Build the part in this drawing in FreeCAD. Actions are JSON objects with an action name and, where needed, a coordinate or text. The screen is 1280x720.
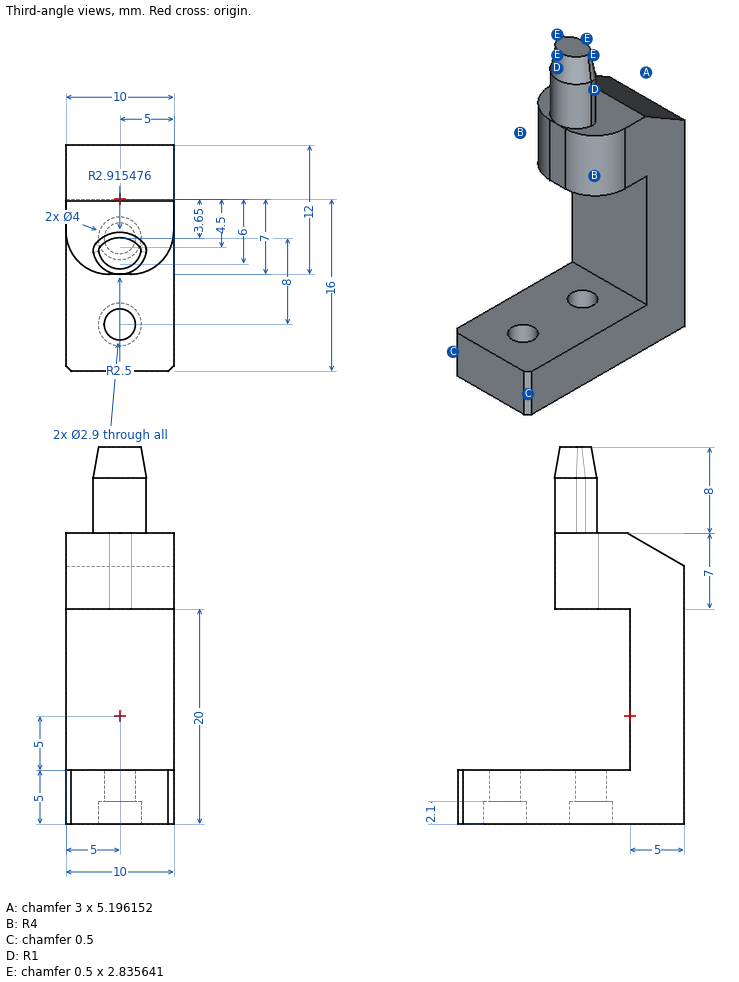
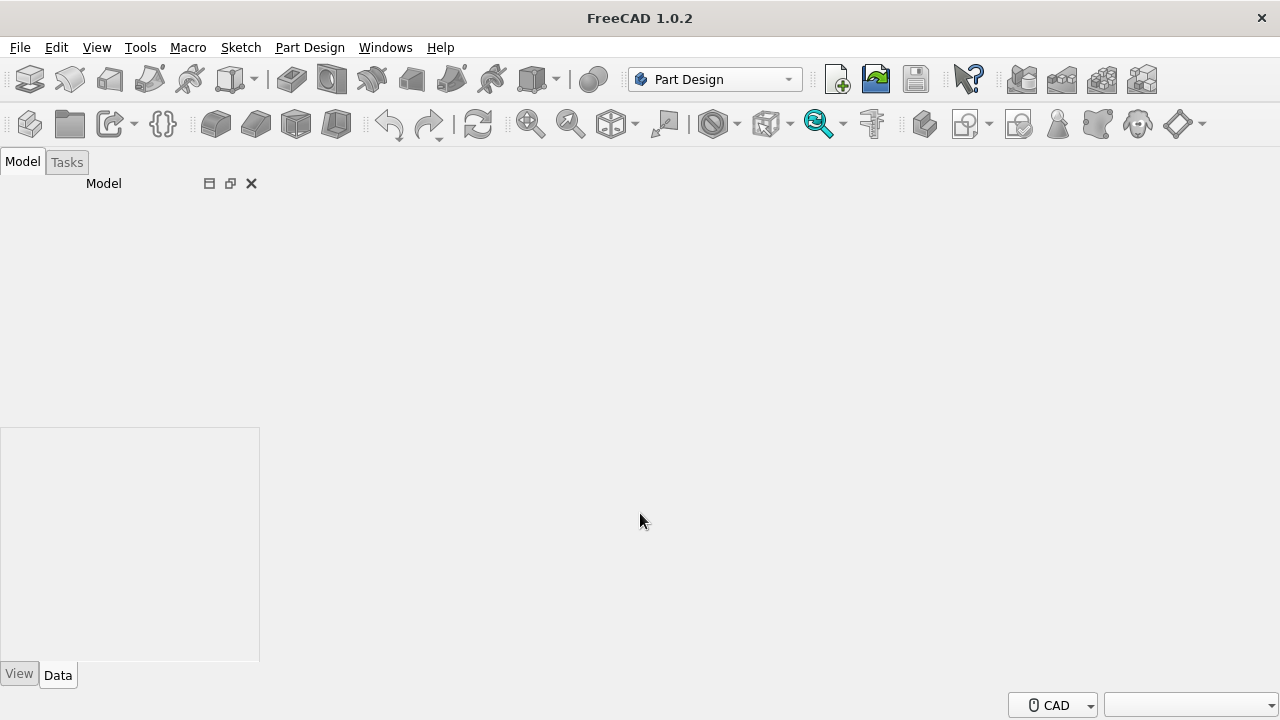
{"action": "key", "text": "ctrl+n"}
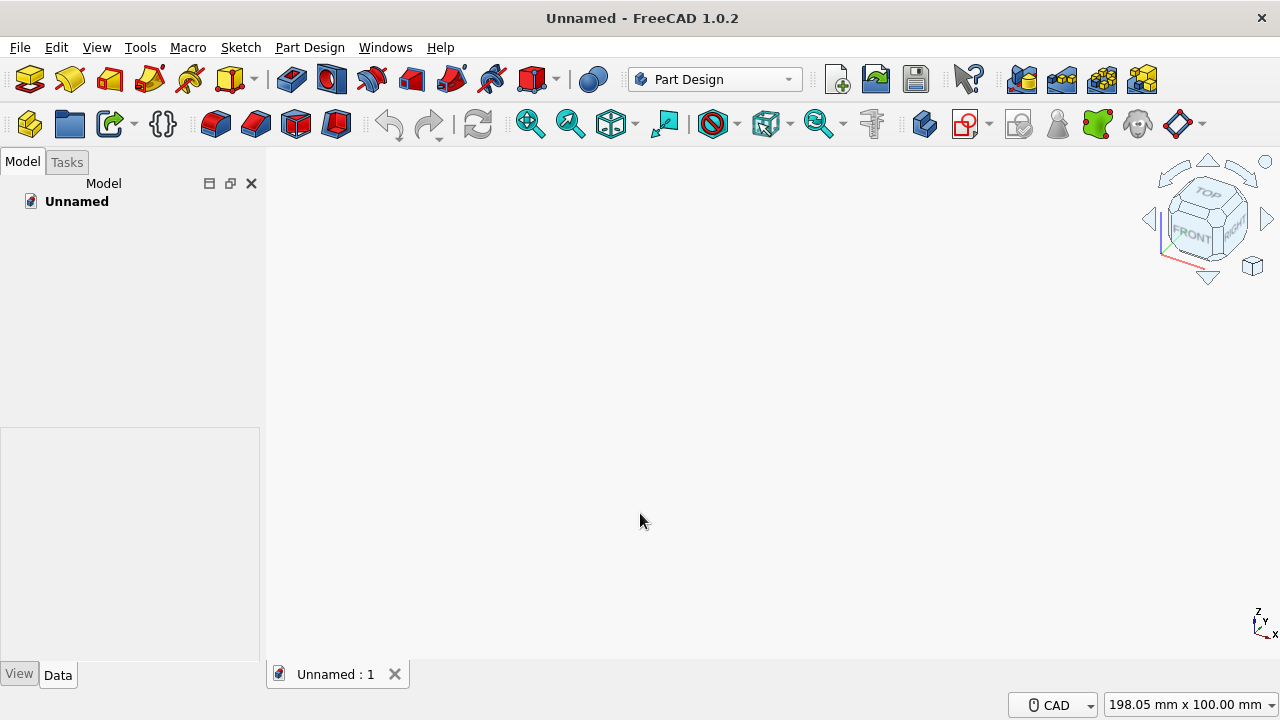
{"action": "left_click", "coordinate": [966, 124]}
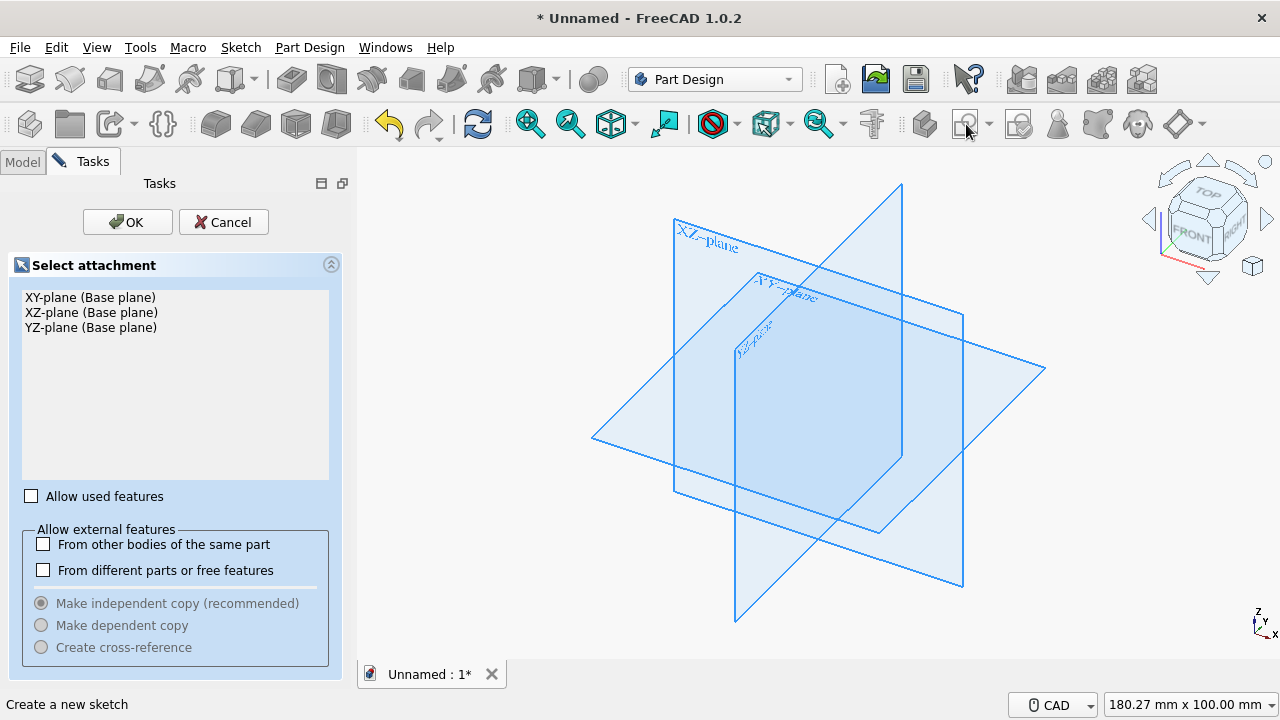
{"action": "left_click", "coordinate": [82, 312]}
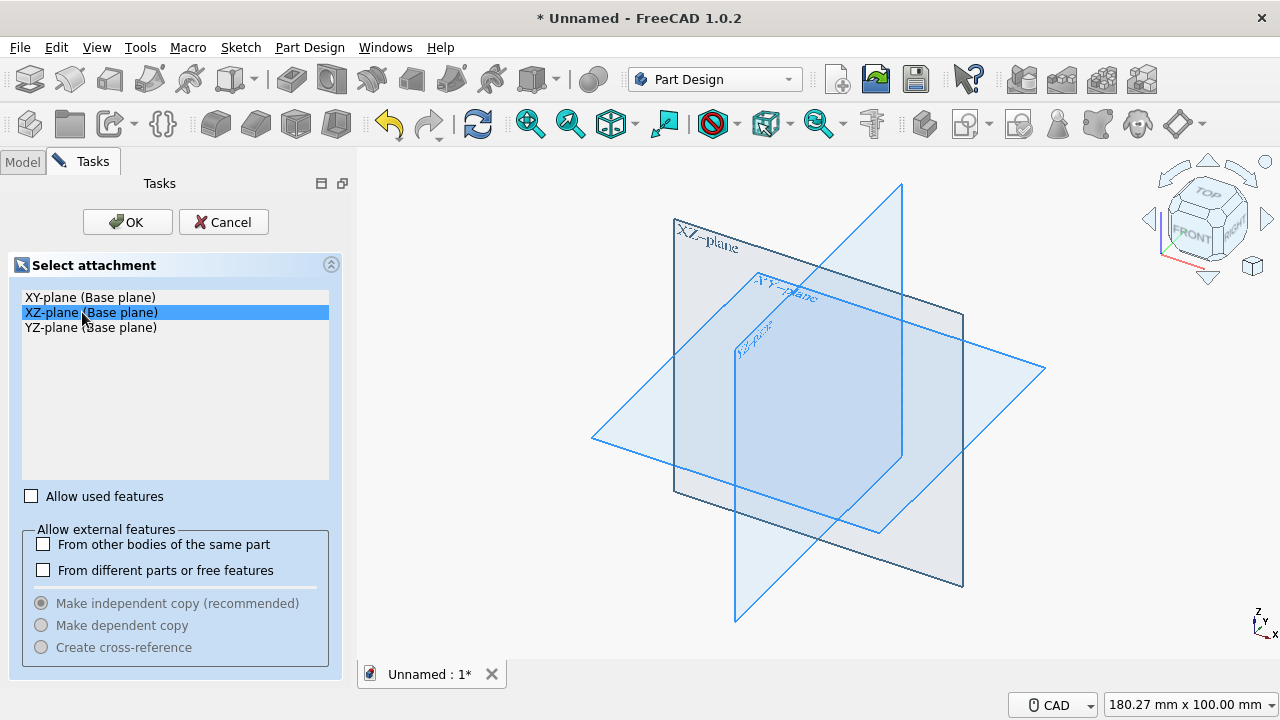
{"action": "left_click", "coordinate": [128, 222]}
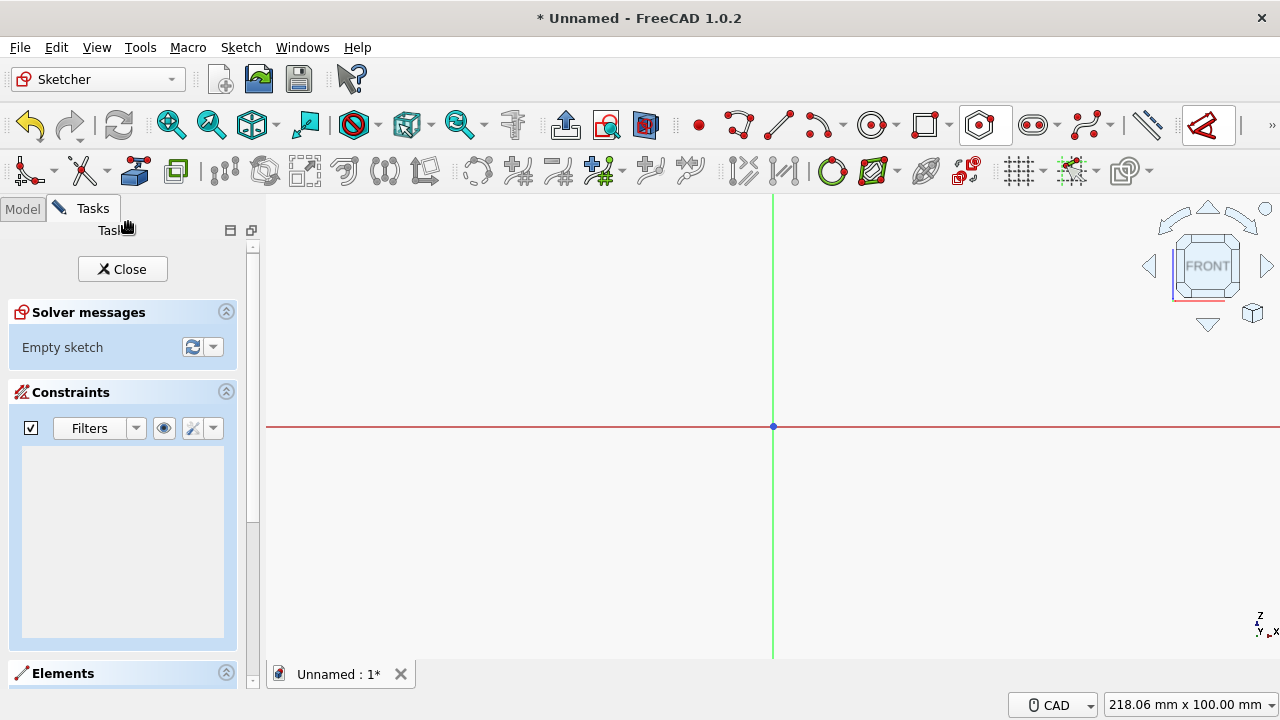
{"action": "scroll", "coordinate": [803, 427], "scroll_direction": "up", "scroll_amount": 6}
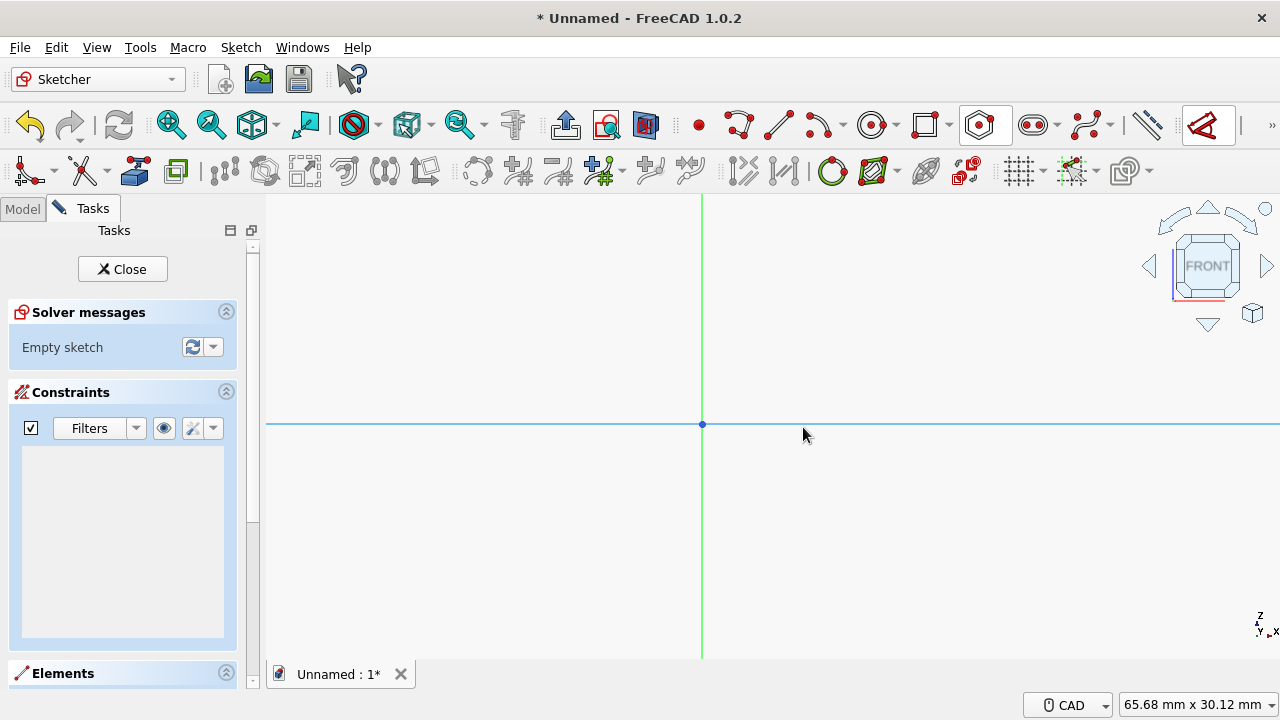
{"action": "key", "text": "g v"}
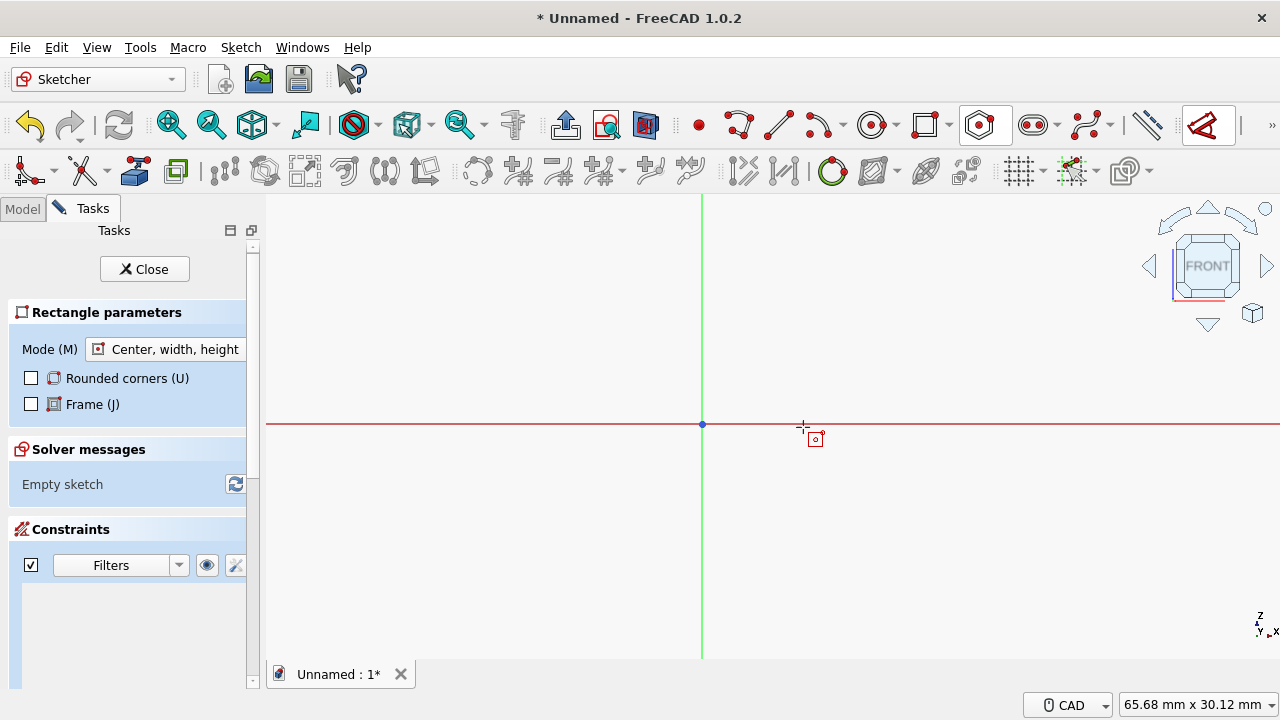
{"action": "left_click", "coordinate": [702, 424]}
{"action": "left_click", "coordinate": [779, 270]}
{"action": "key", "text": "Escape"}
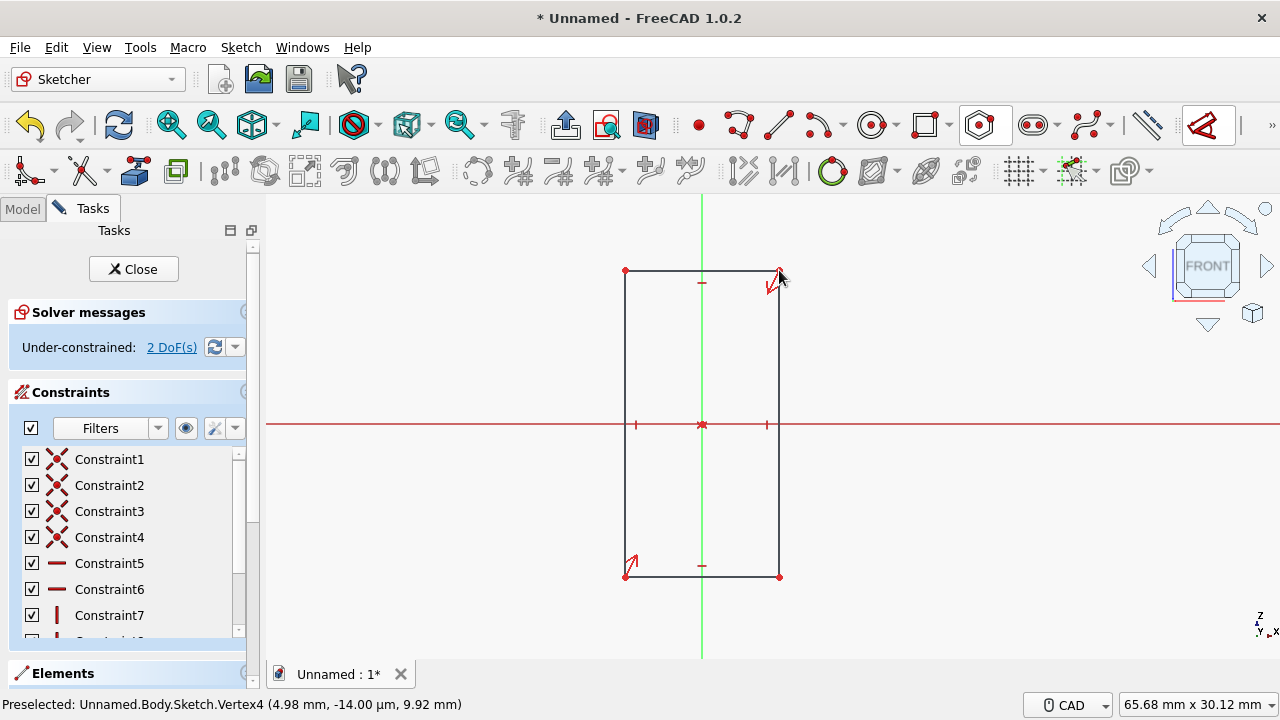
{"action": "key", "text": "d"}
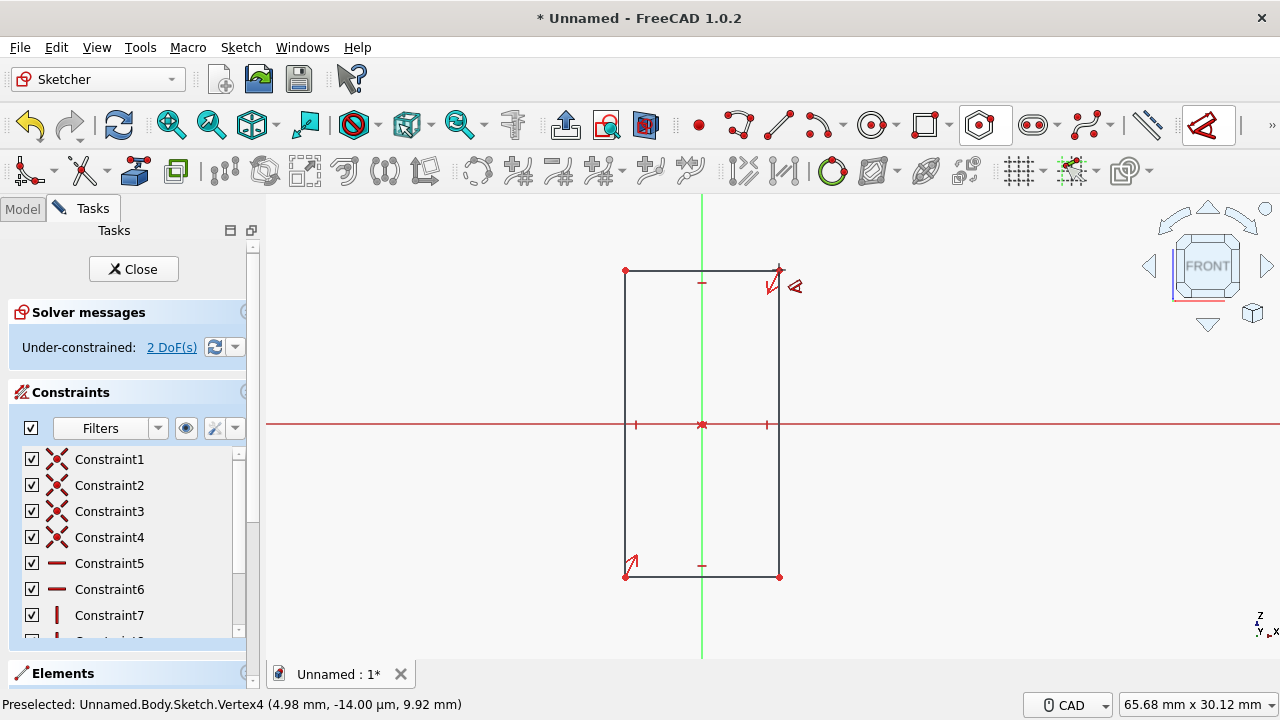
{"action": "left_click", "coordinate": [671, 577]}
{"action": "left_click", "coordinate": [667, 611]}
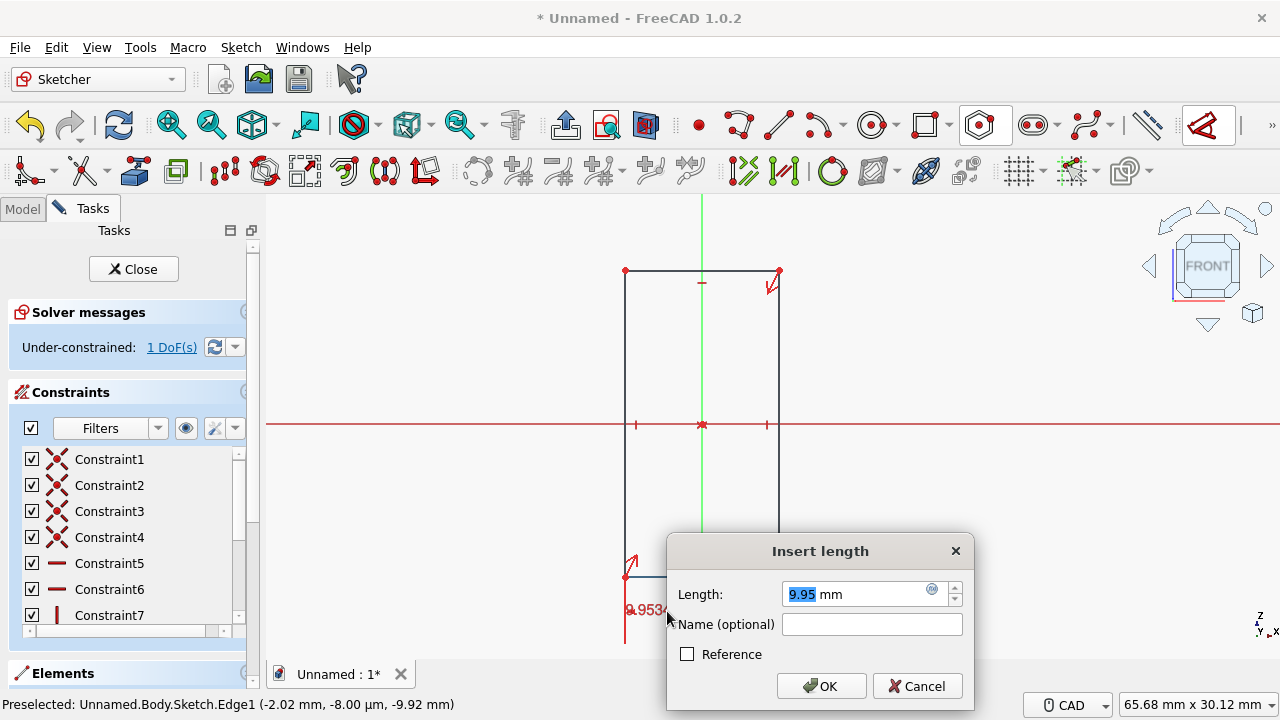
{"action": "type", "text": "10"}
{"action": "key", "text": "Return"}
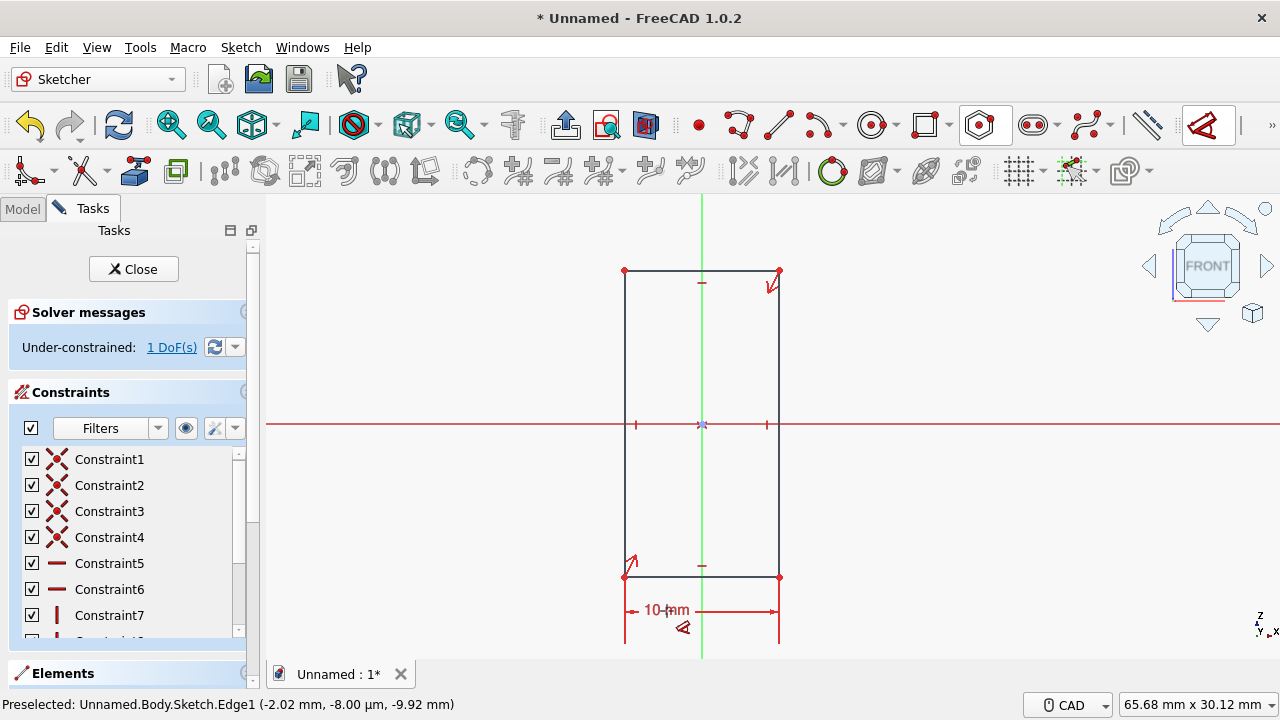
{"action": "left_click", "coordinate": [779, 485]}
{"action": "left_click", "coordinate": [813, 354]}